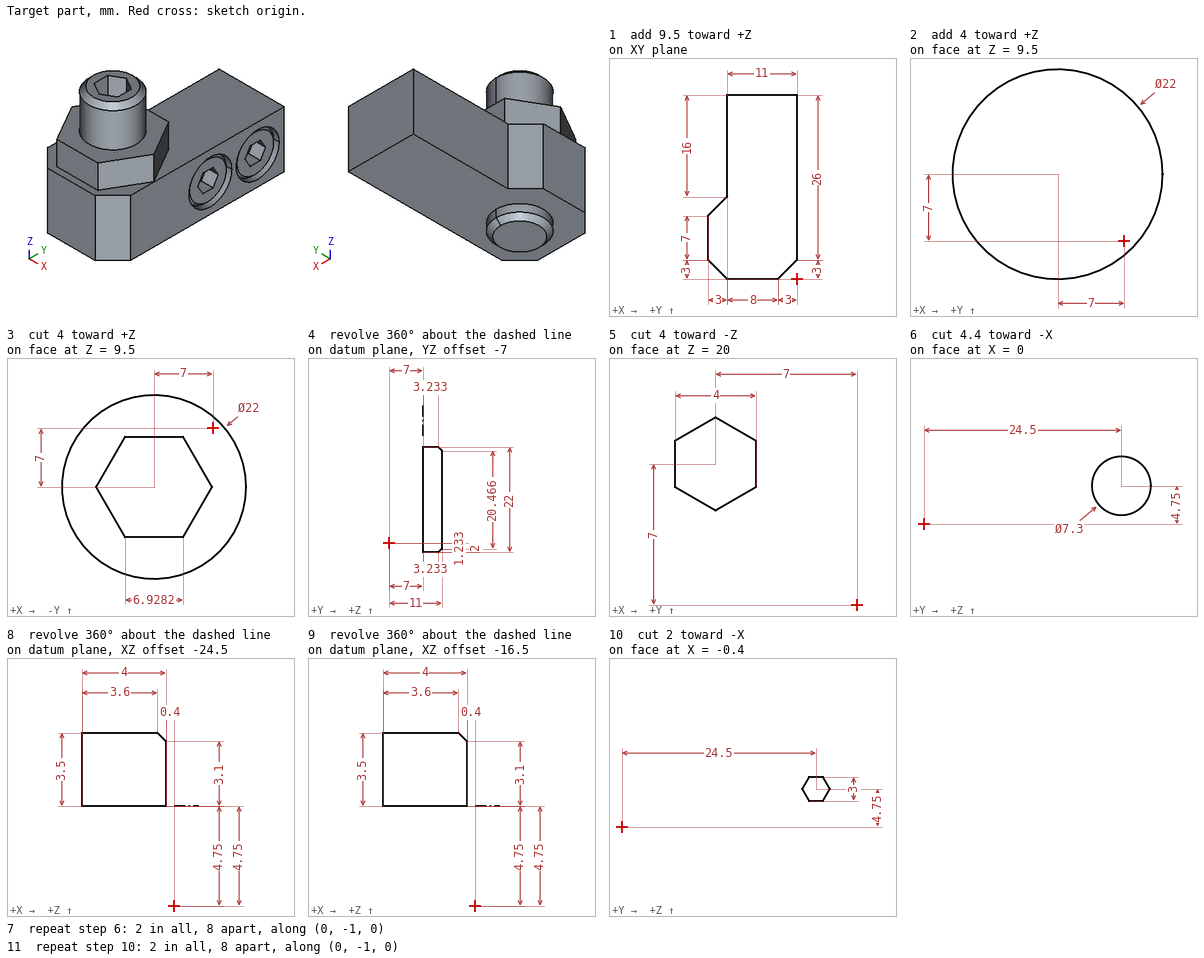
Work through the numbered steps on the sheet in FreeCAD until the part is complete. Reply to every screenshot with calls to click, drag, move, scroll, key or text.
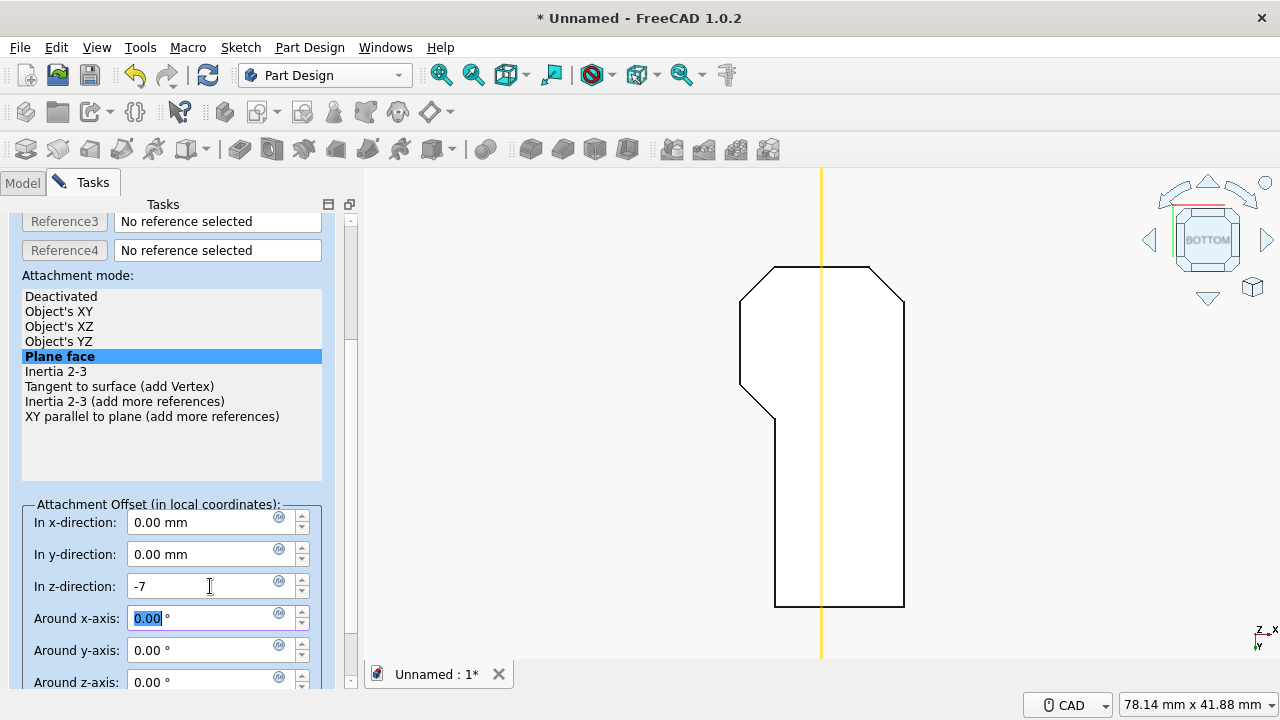
scroll(351, 451, up, 4)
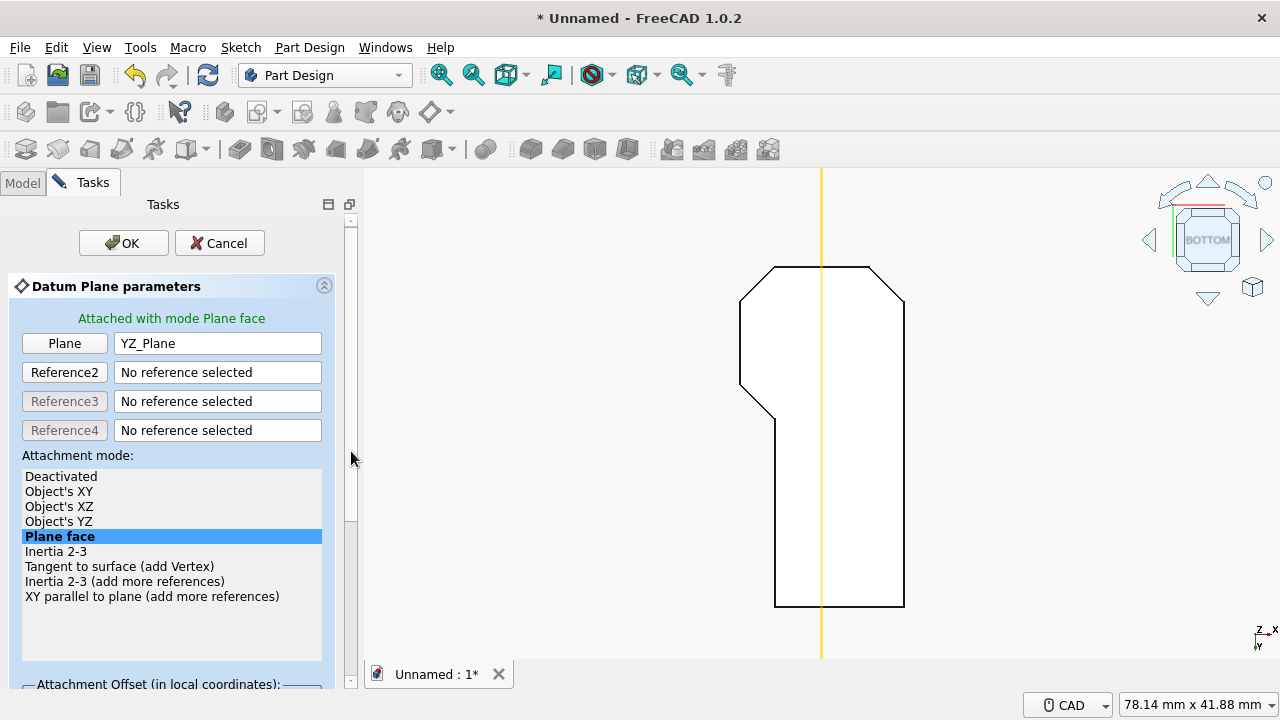
click(124, 243)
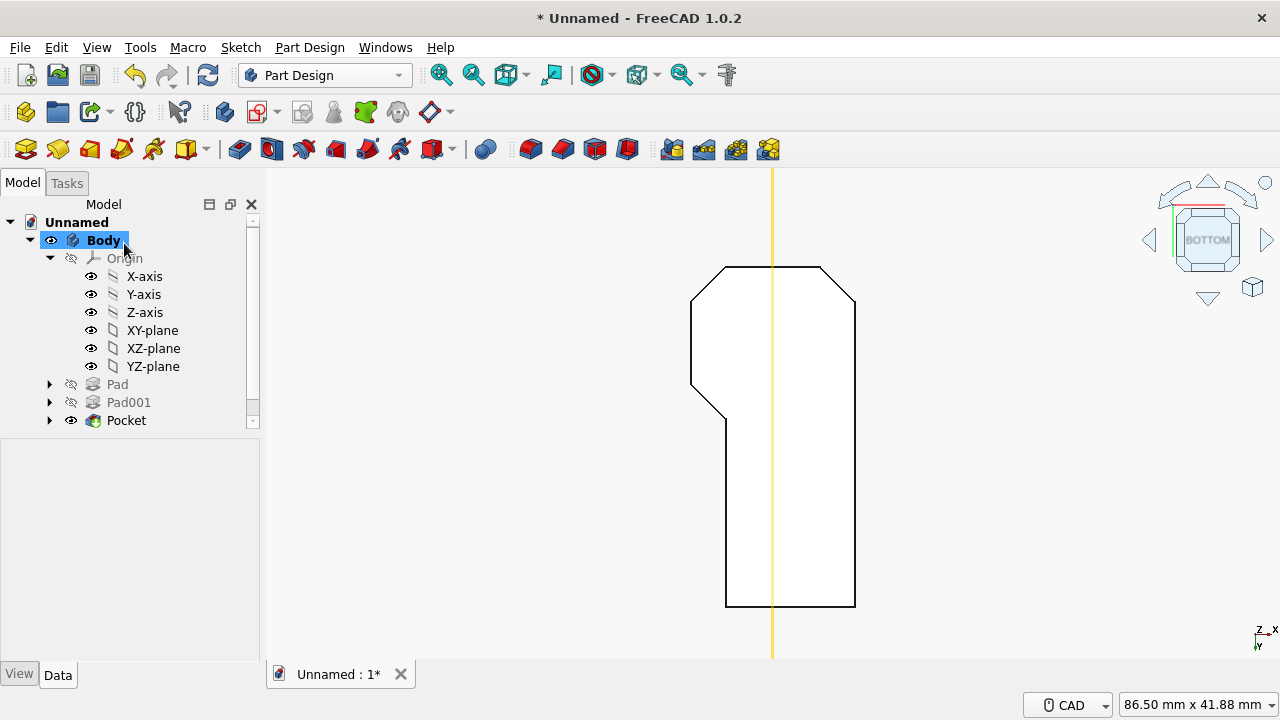
scroll(100, 326, down, 3)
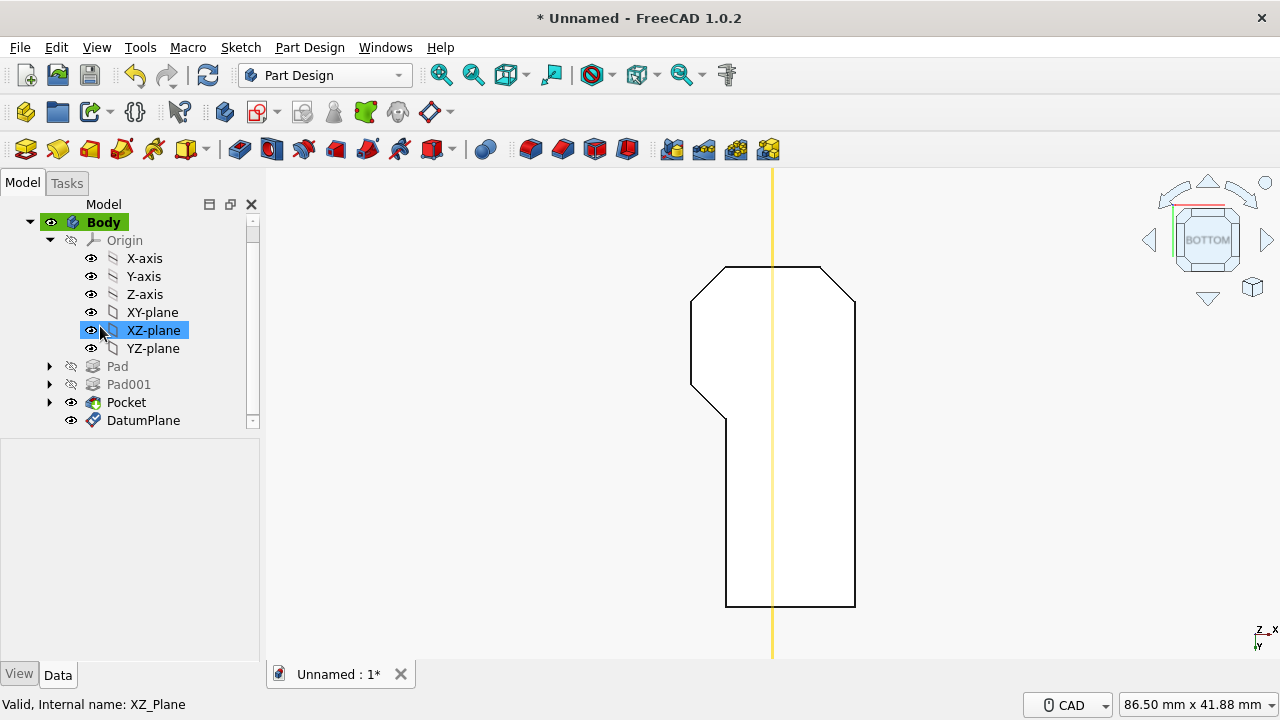
click(116, 420)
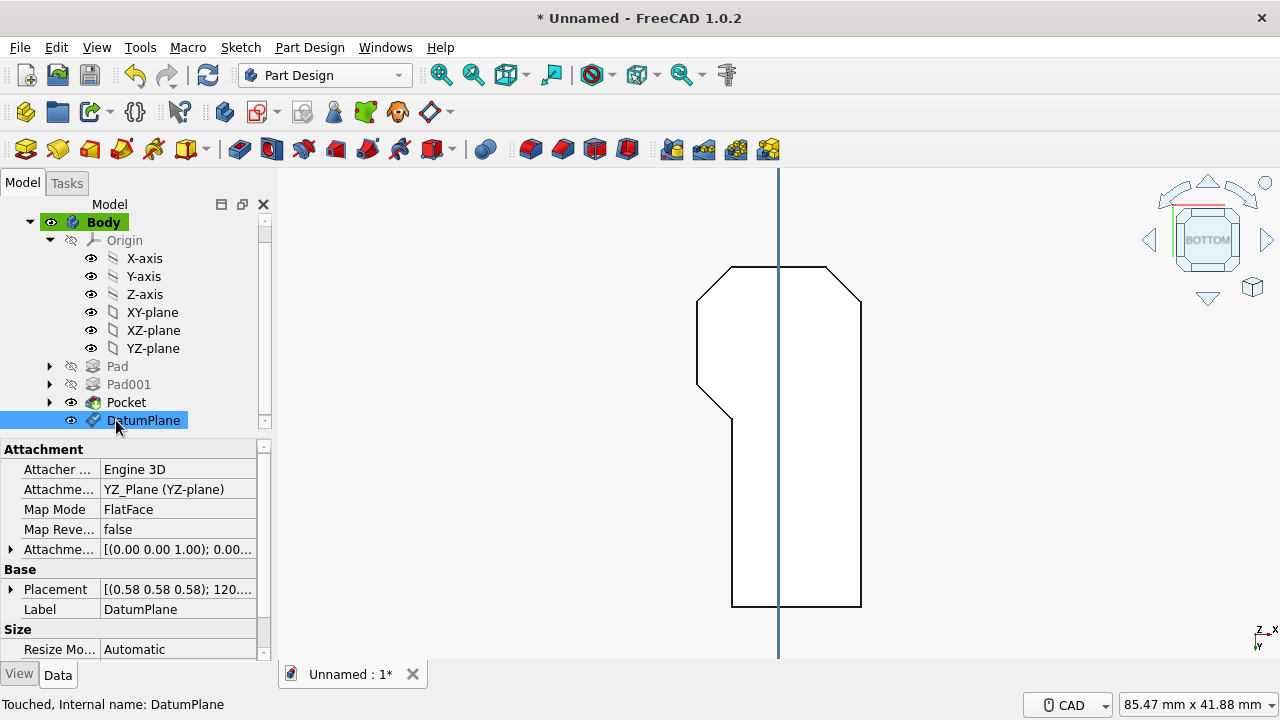
click(258, 112)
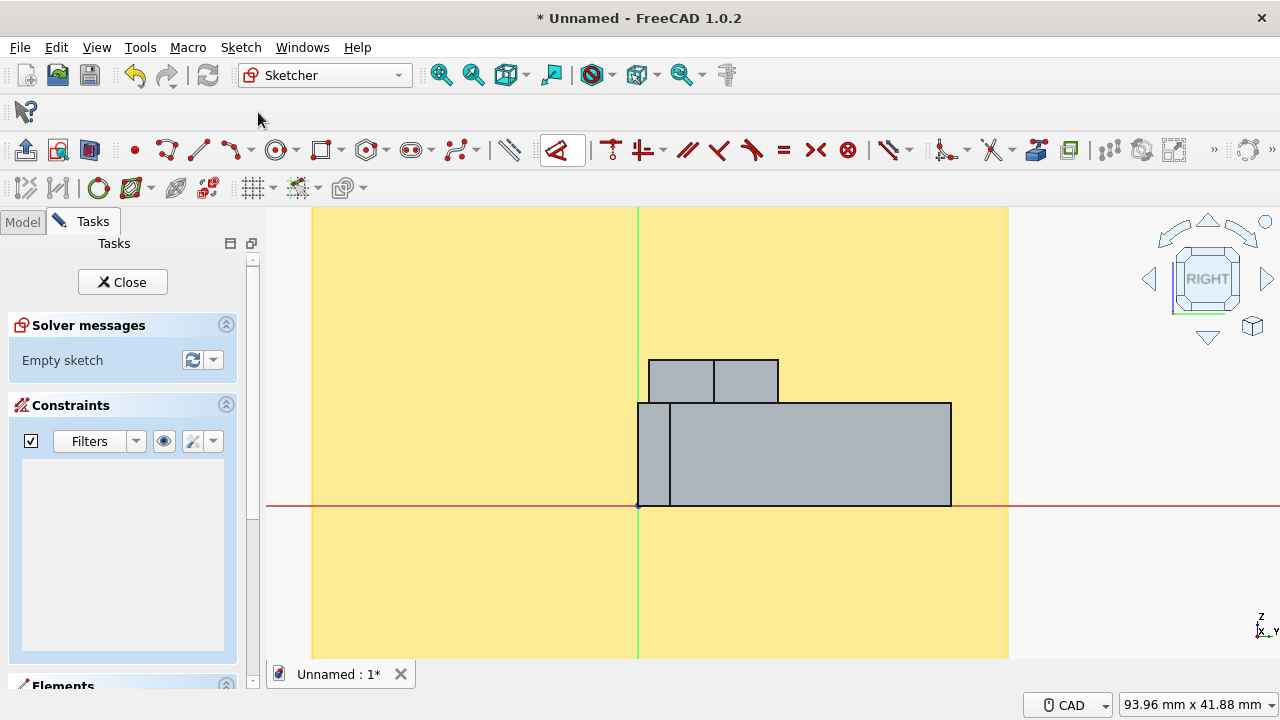
key(q)
key(s)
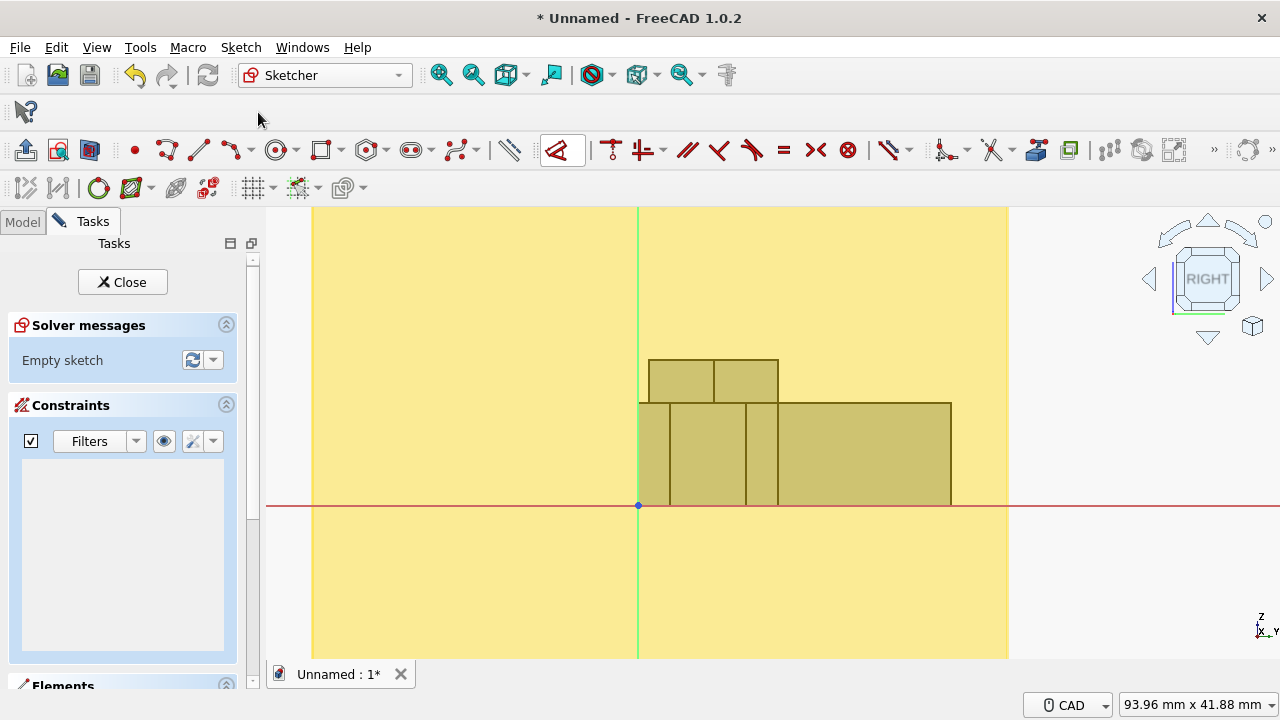
scroll(736, 631, down, 1)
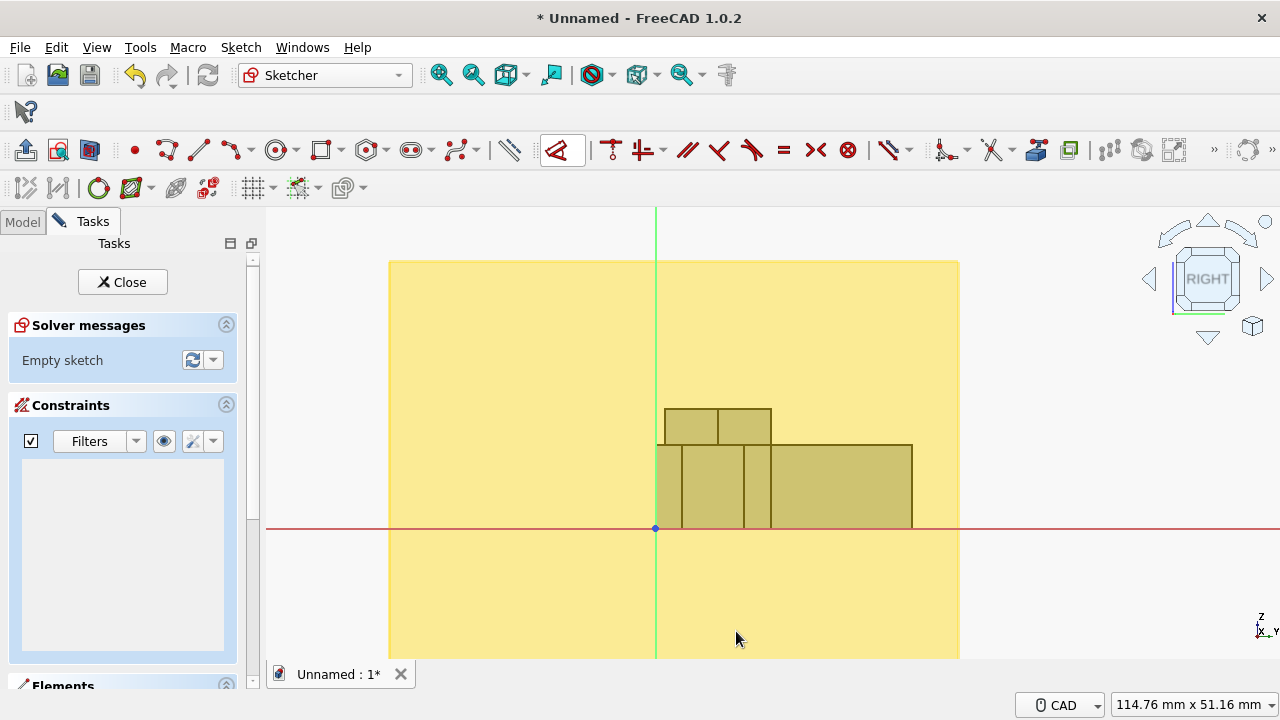
click(168, 150)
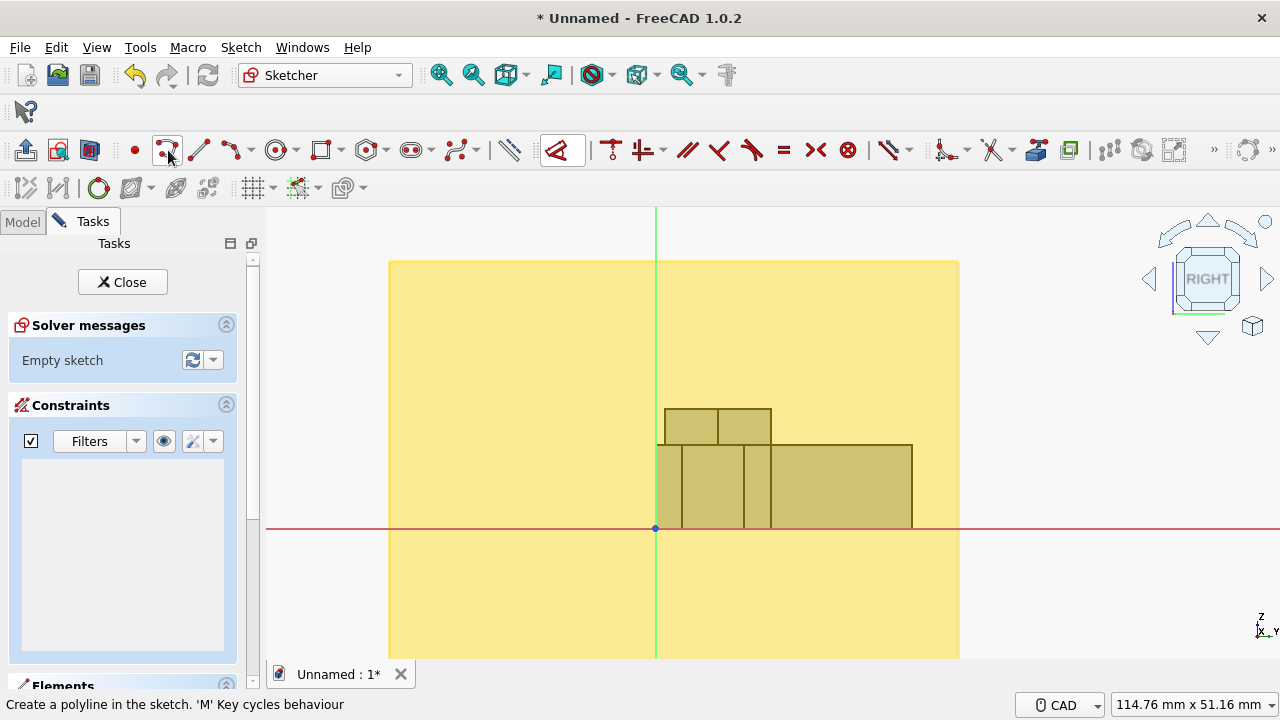
click(718, 546)
click(746, 546)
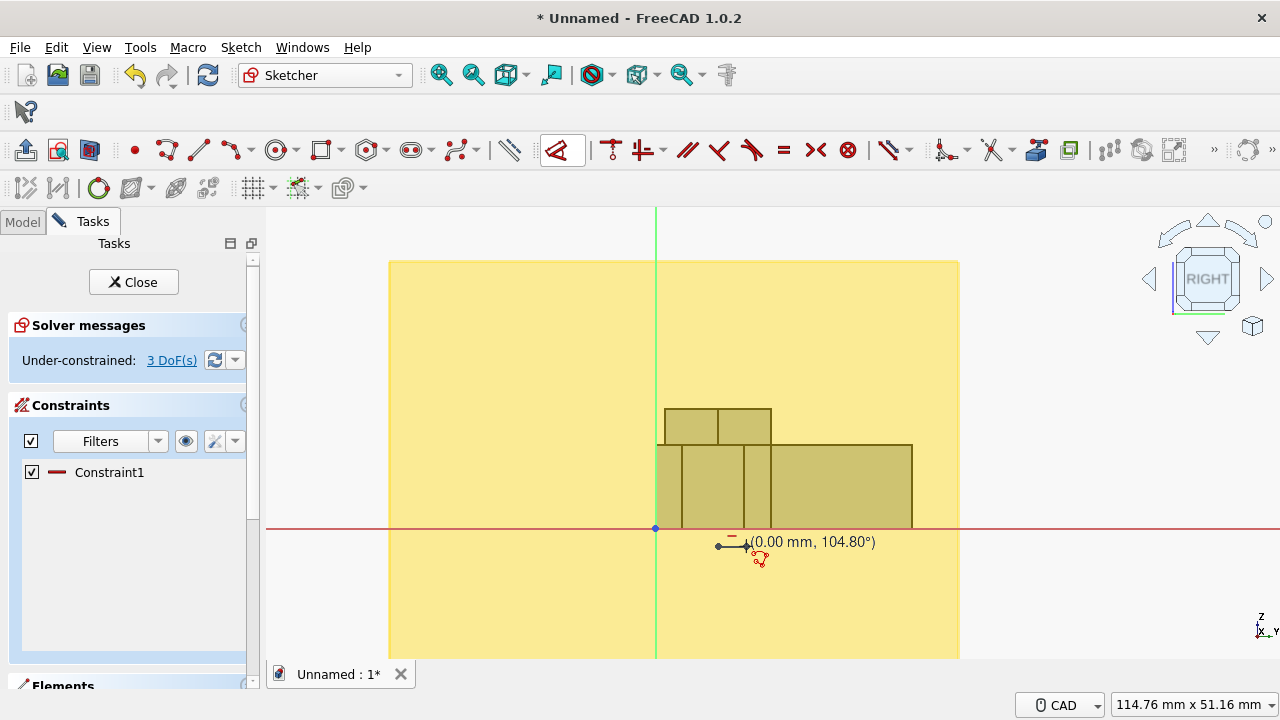
scroll(753, 540, up, 3)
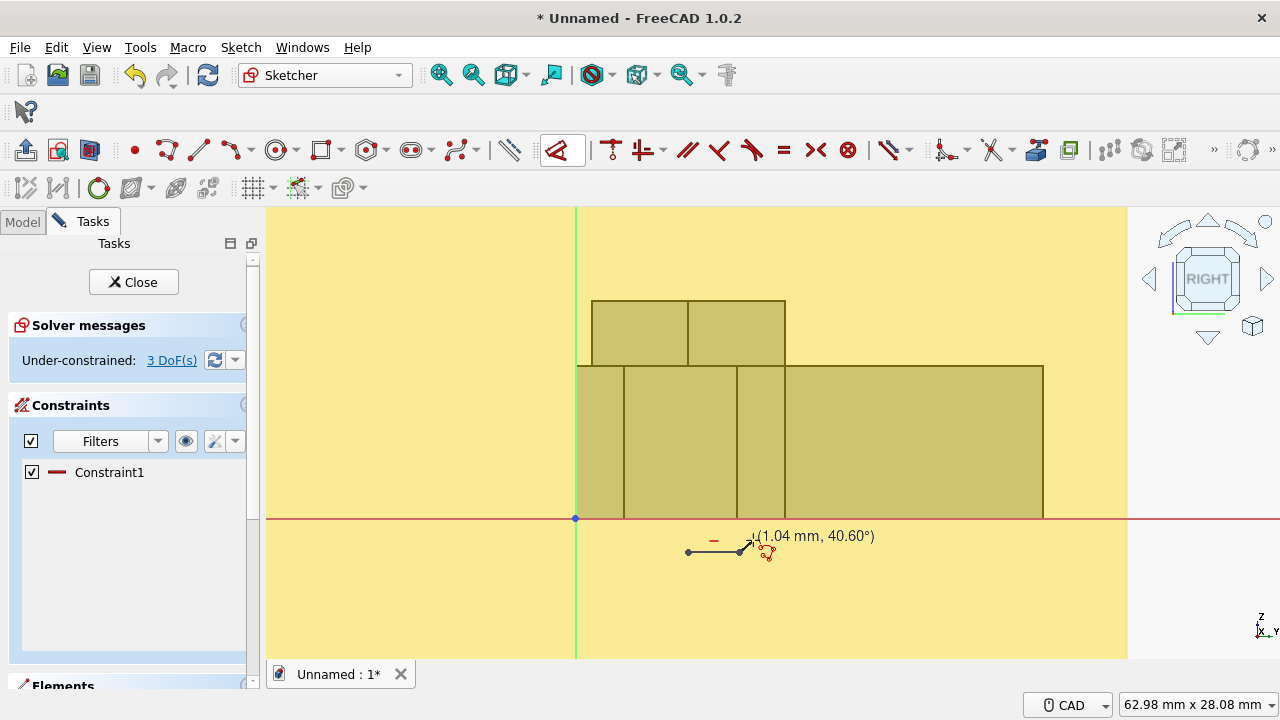
click(753, 539)